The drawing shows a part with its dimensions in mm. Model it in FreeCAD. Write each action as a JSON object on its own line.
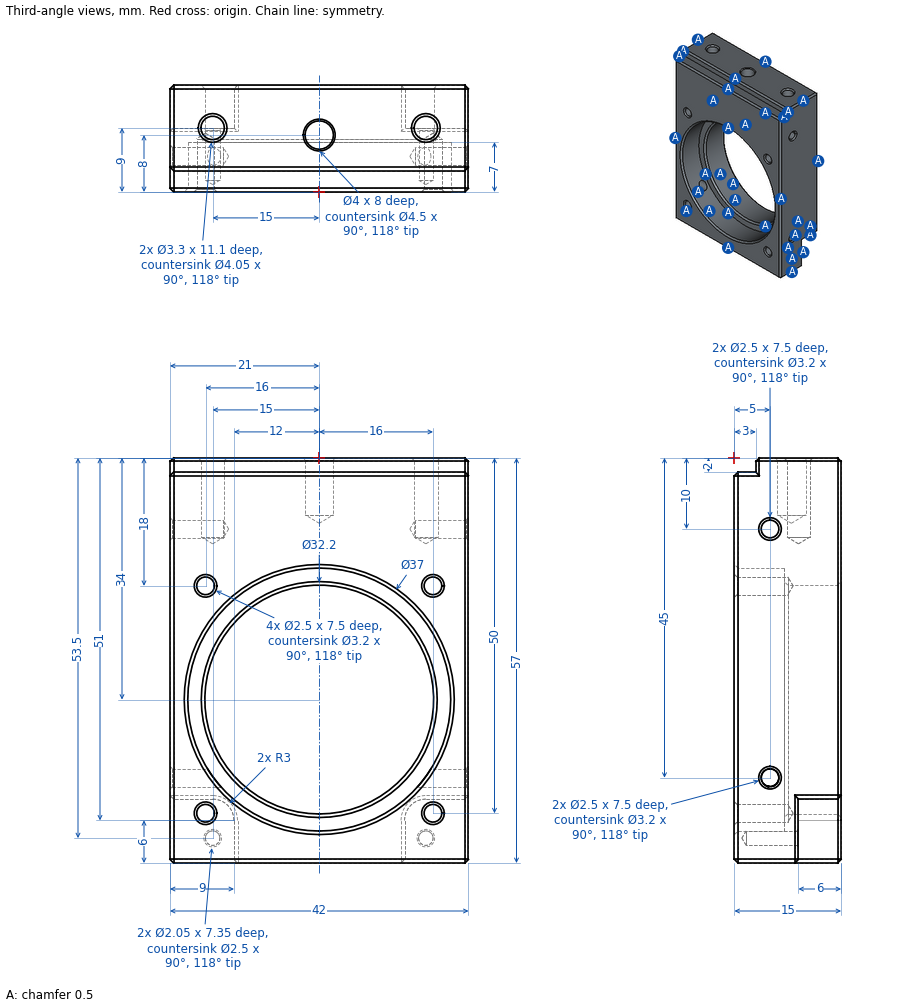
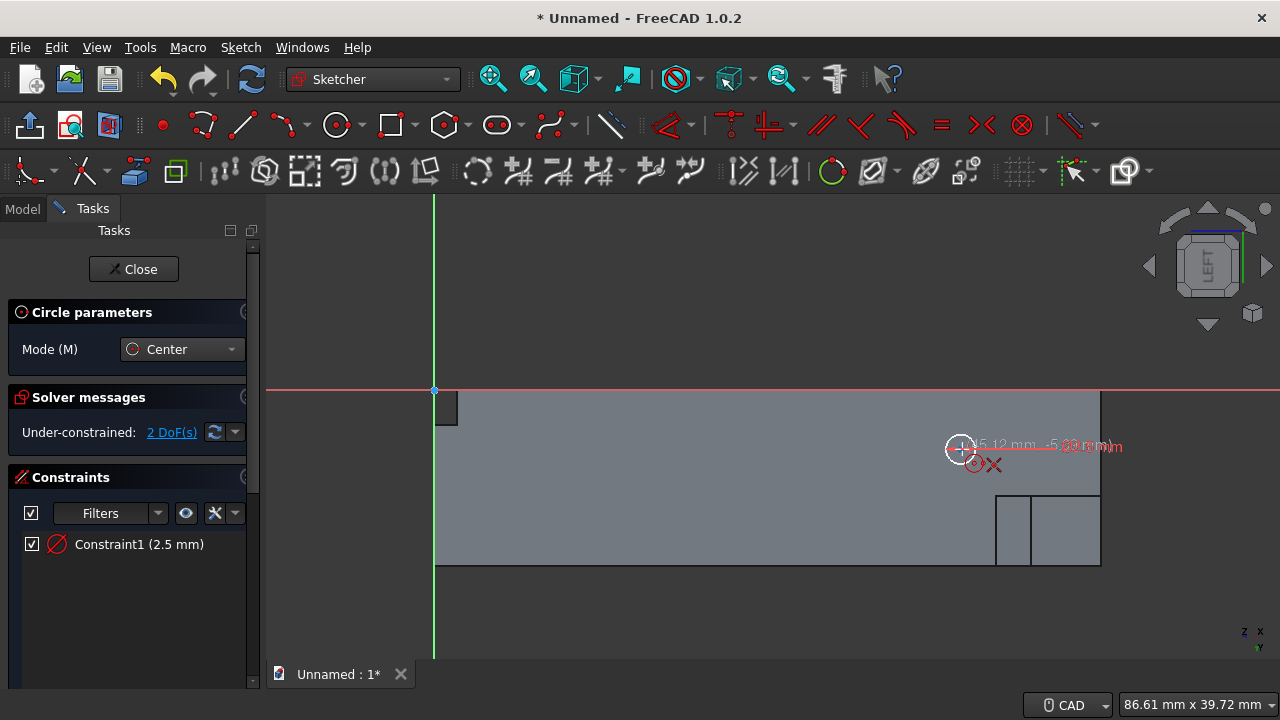
{"action": "scroll", "coordinate": [551, 449], "scroll_direction": "up", "scroll_amount": 3}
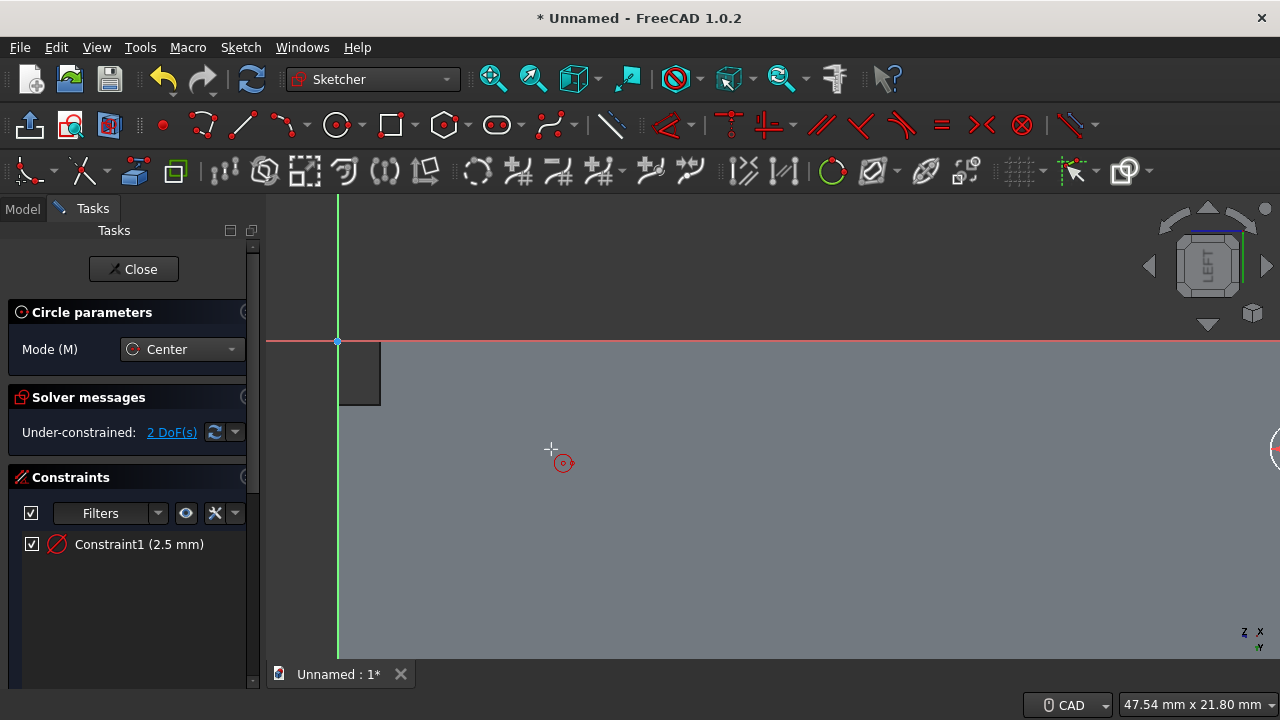
{"action": "left_click", "coordinate": [551, 448]}
{"action": "mouse_move", "coordinate": [570, 429]}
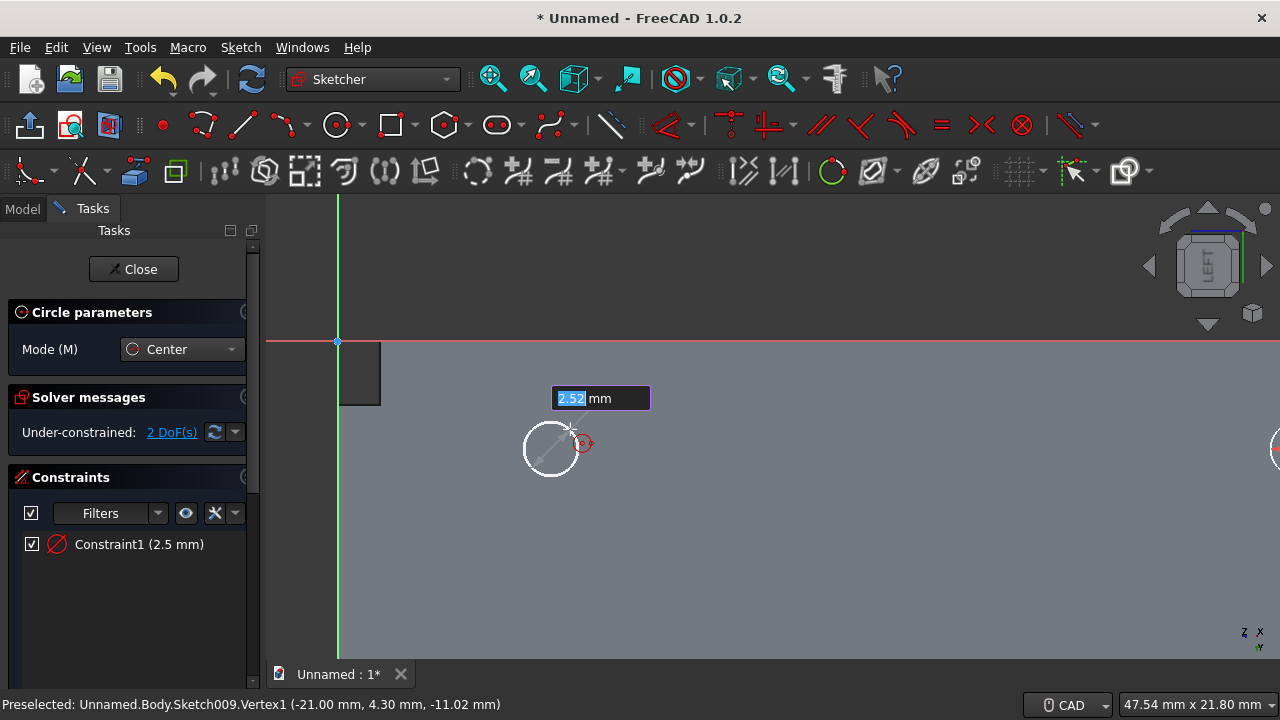
{"action": "type", "text": "2.5"}
{"action": "key", "text": "Return"}
{"action": "key", "text": "Escape"}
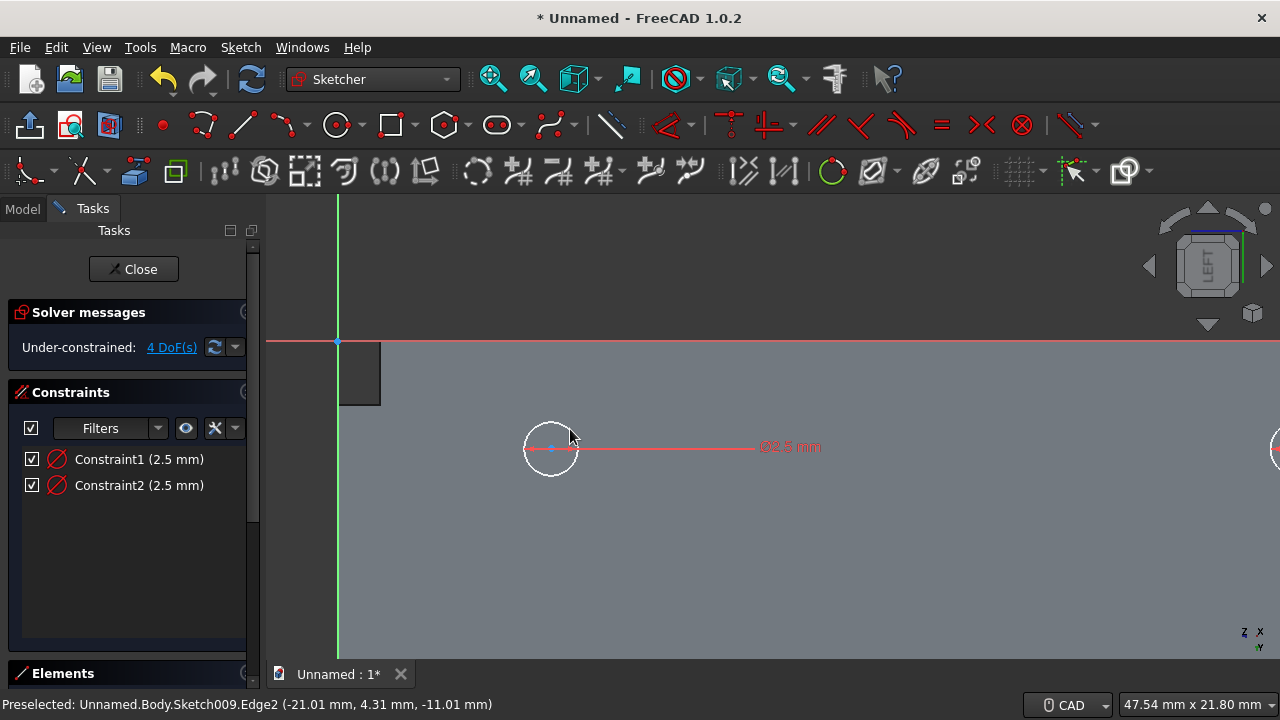
{"action": "left_click", "coordinate": [666, 126]}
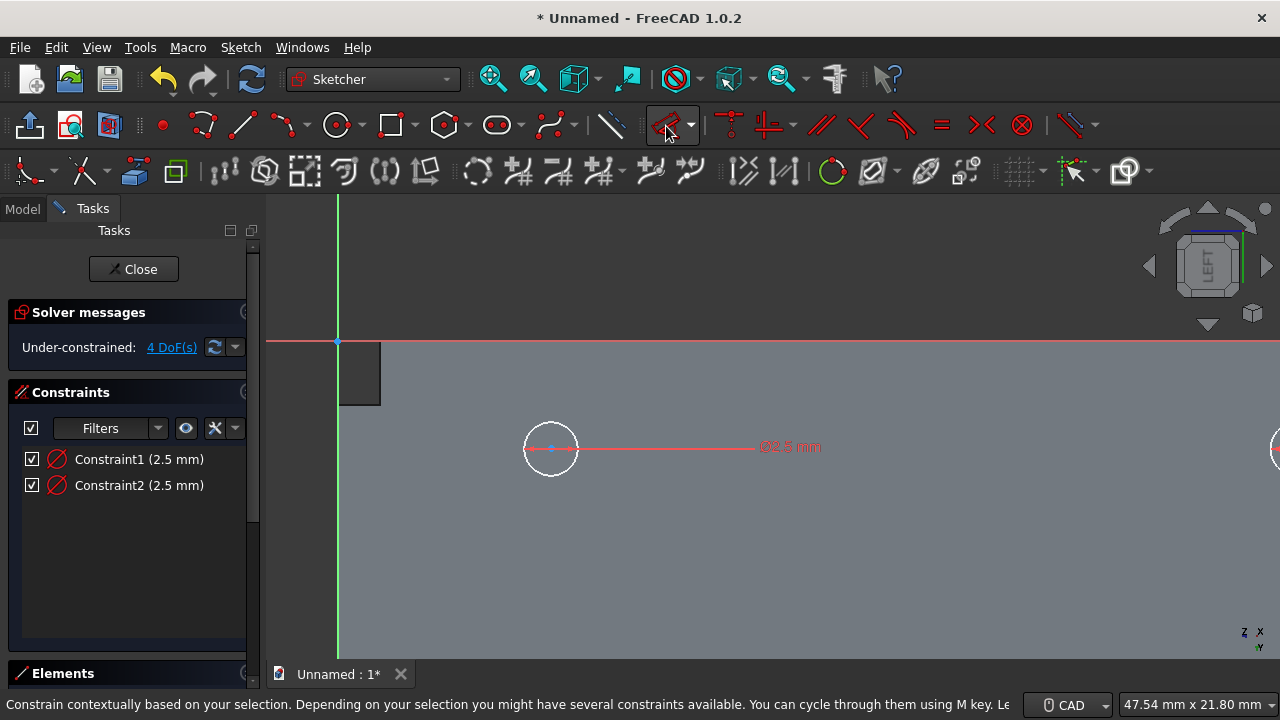
{"action": "scroll", "coordinate": [551, 449], "scroll_direction": "down", "scroll_amount": 3}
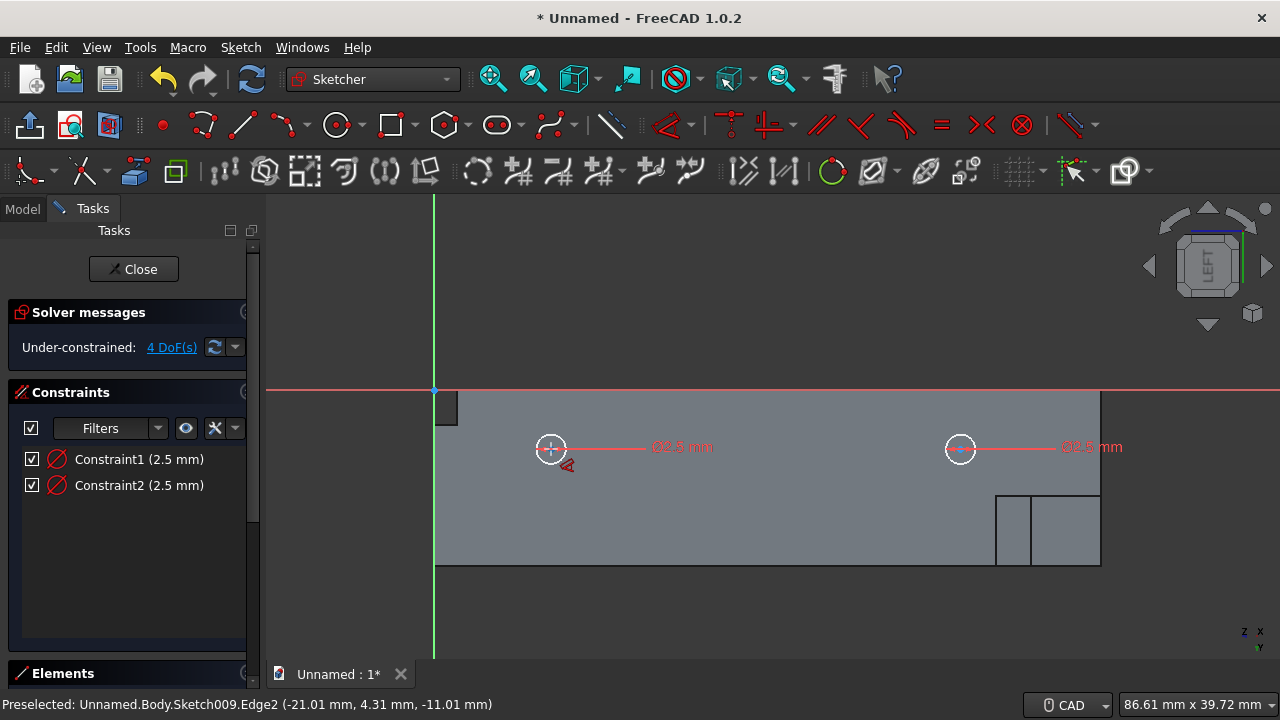
{"action": "left_click", "coordinate": [961, 449]}
{"action": "left_click", "coordinate": [400, 420]}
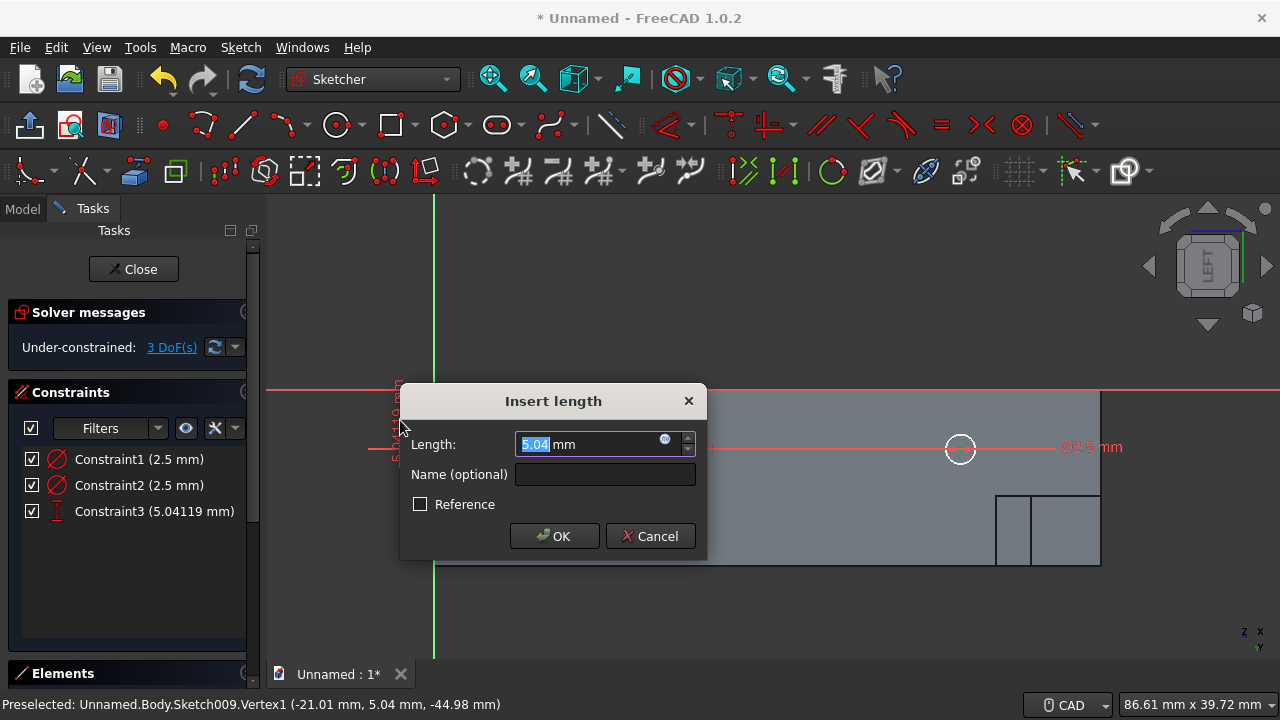
{"action": "type", "text": "5"}
{"action": "key", "text": "Return"}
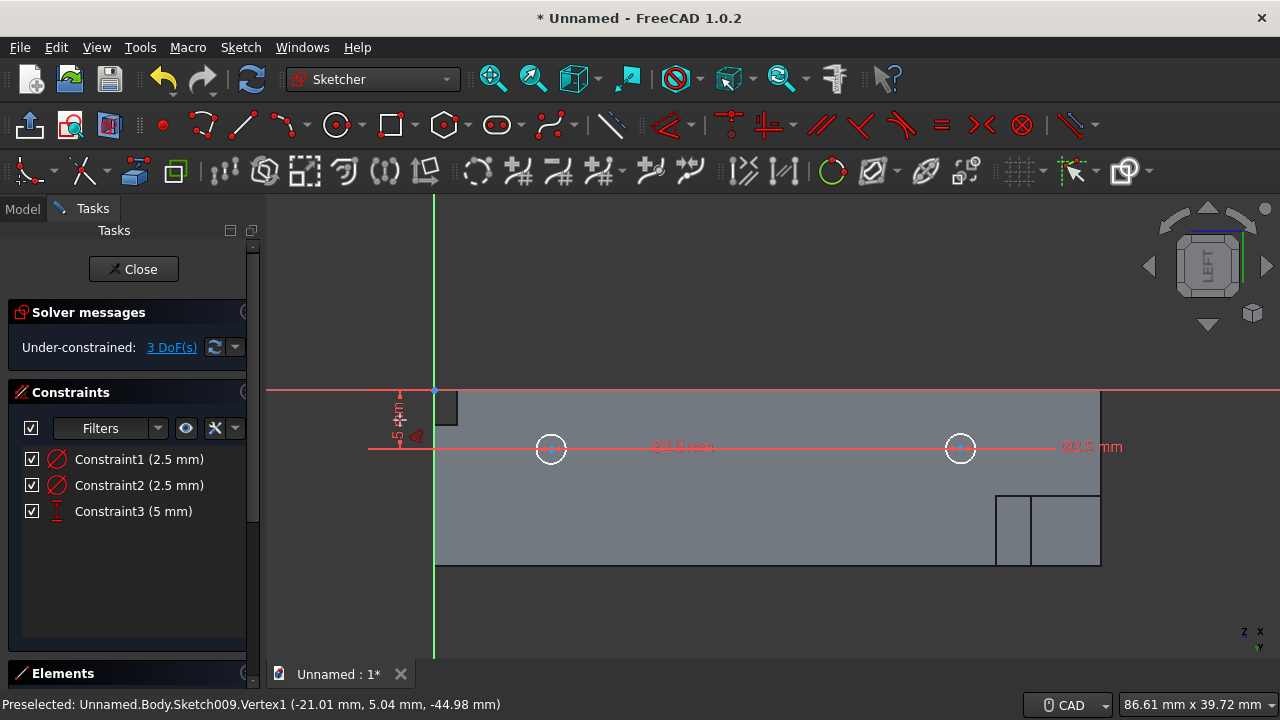
{"action": "left_click", "coordinate": [551, 449]}
{"action": "left_click", "coordinate": [400, 440]}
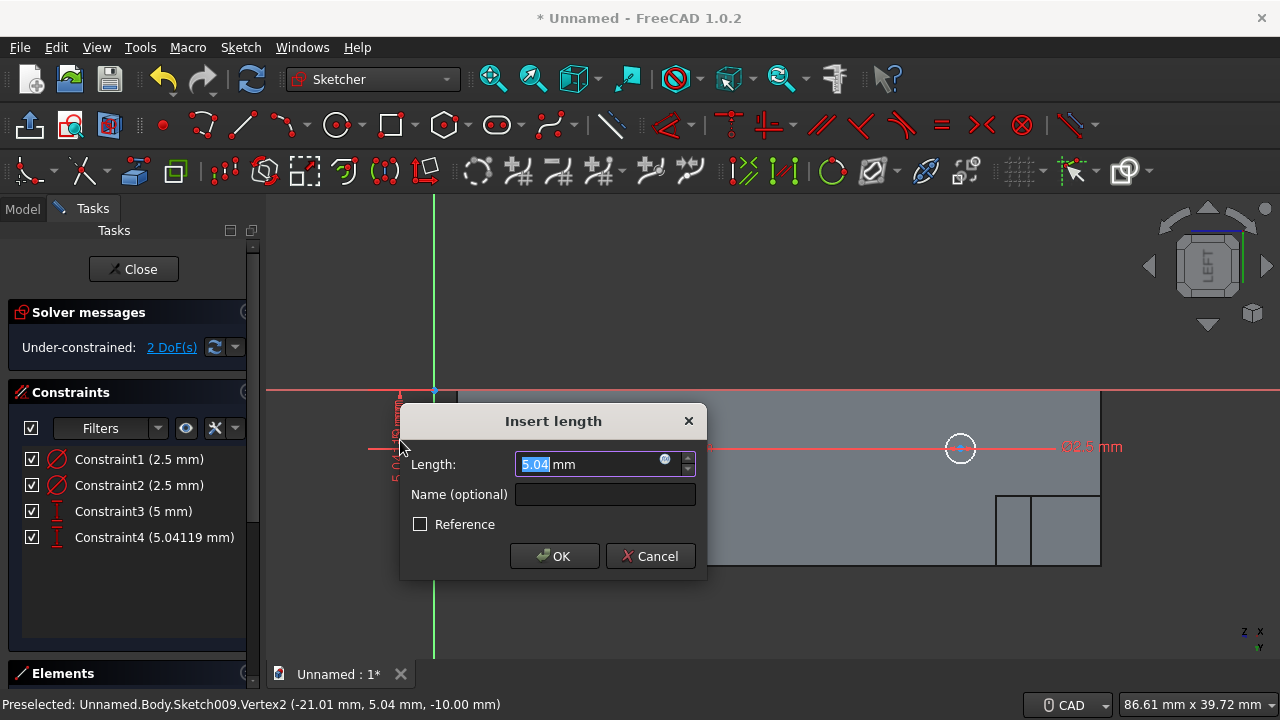
{"action": "type", "text": "5"}
{"action": "key", "text": "Return"}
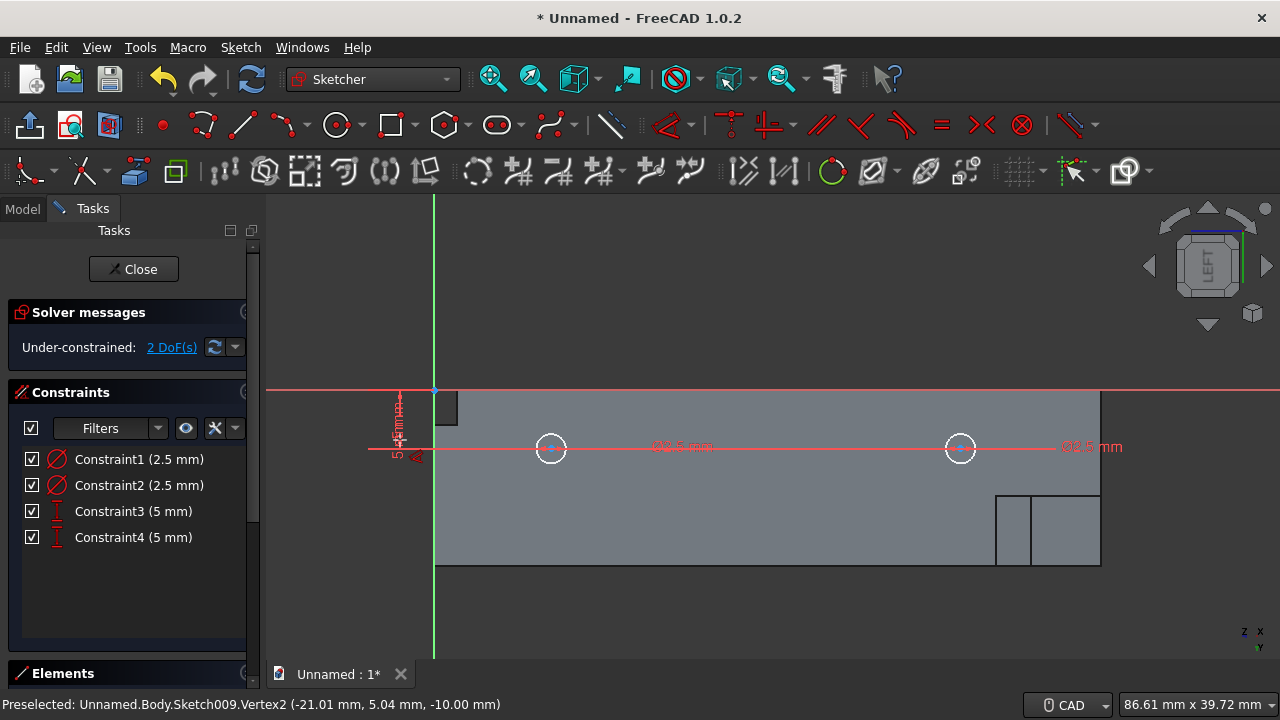
{"action": "left_click", "coordinate": [961, 449]}
{"action": "left_click", "coordinate": [697, 356]}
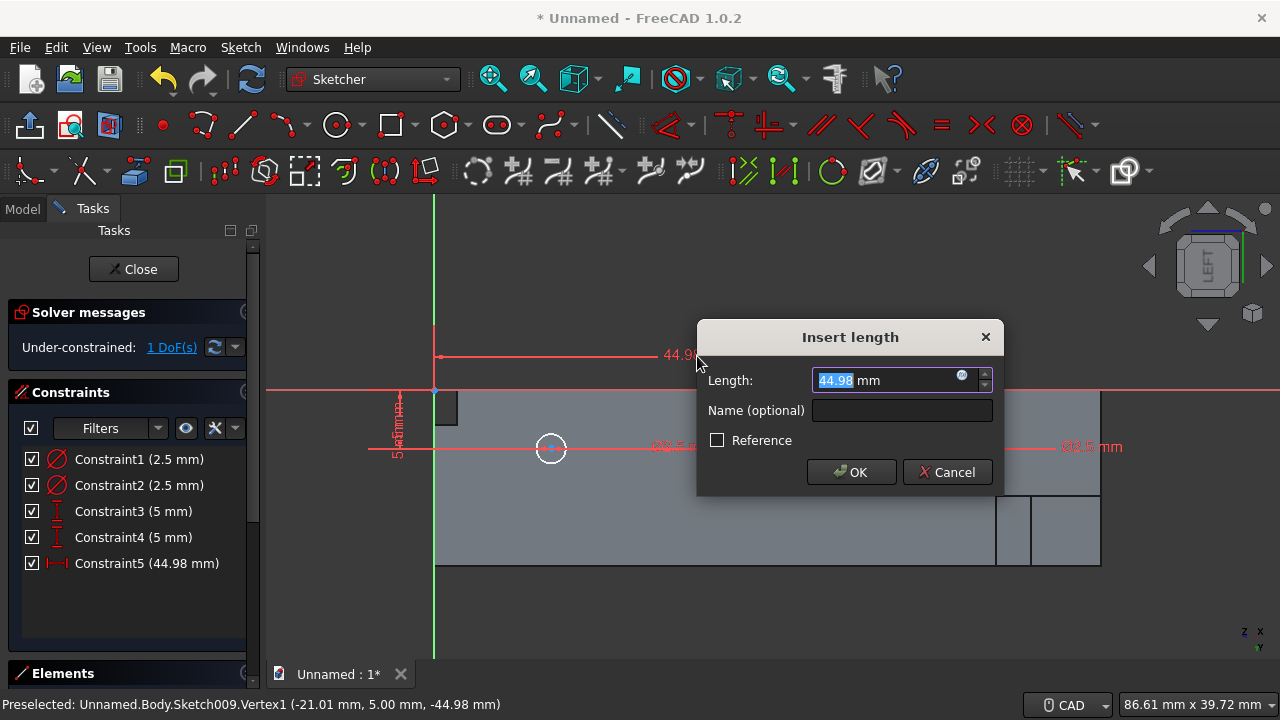
{"action": "type", "text": "45"}
{"action": "key", "text": "Return"}